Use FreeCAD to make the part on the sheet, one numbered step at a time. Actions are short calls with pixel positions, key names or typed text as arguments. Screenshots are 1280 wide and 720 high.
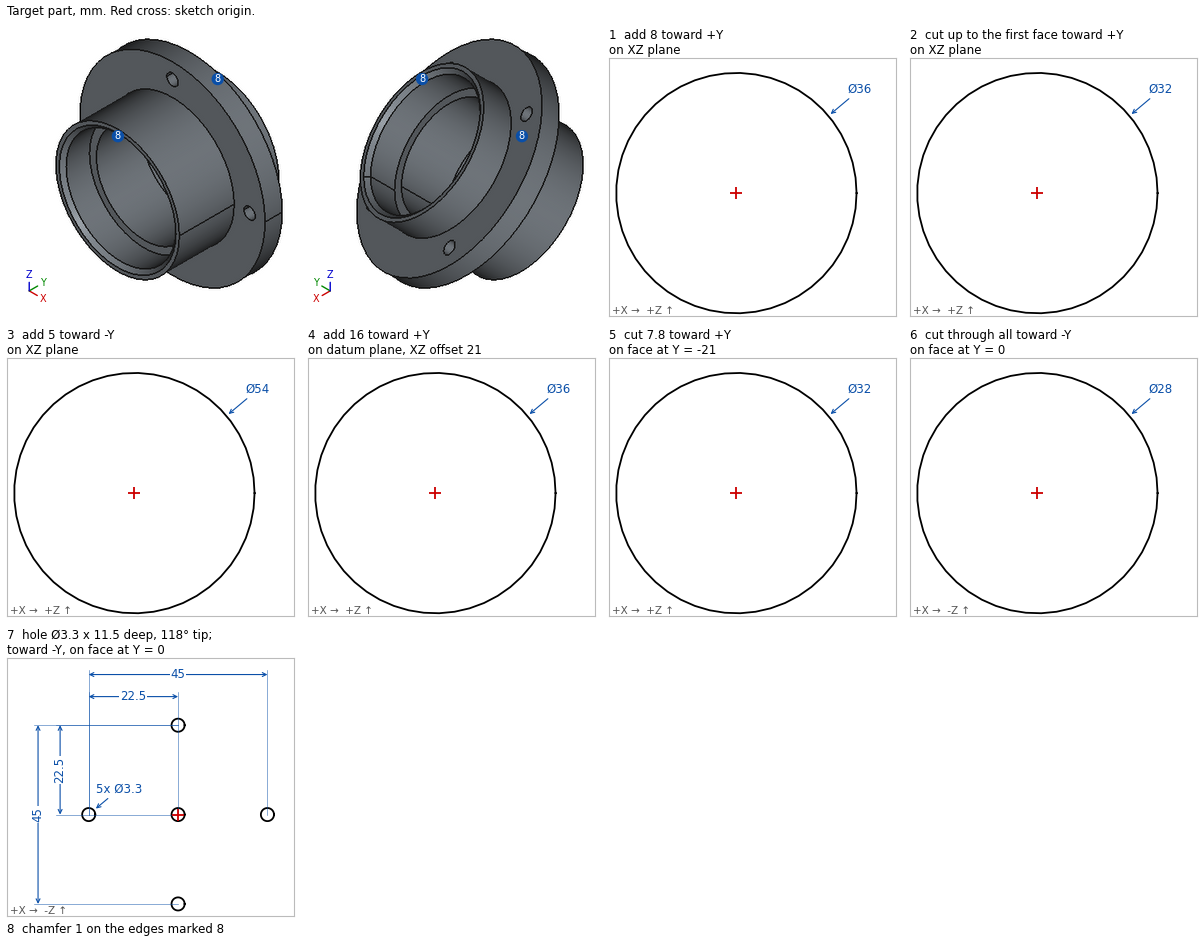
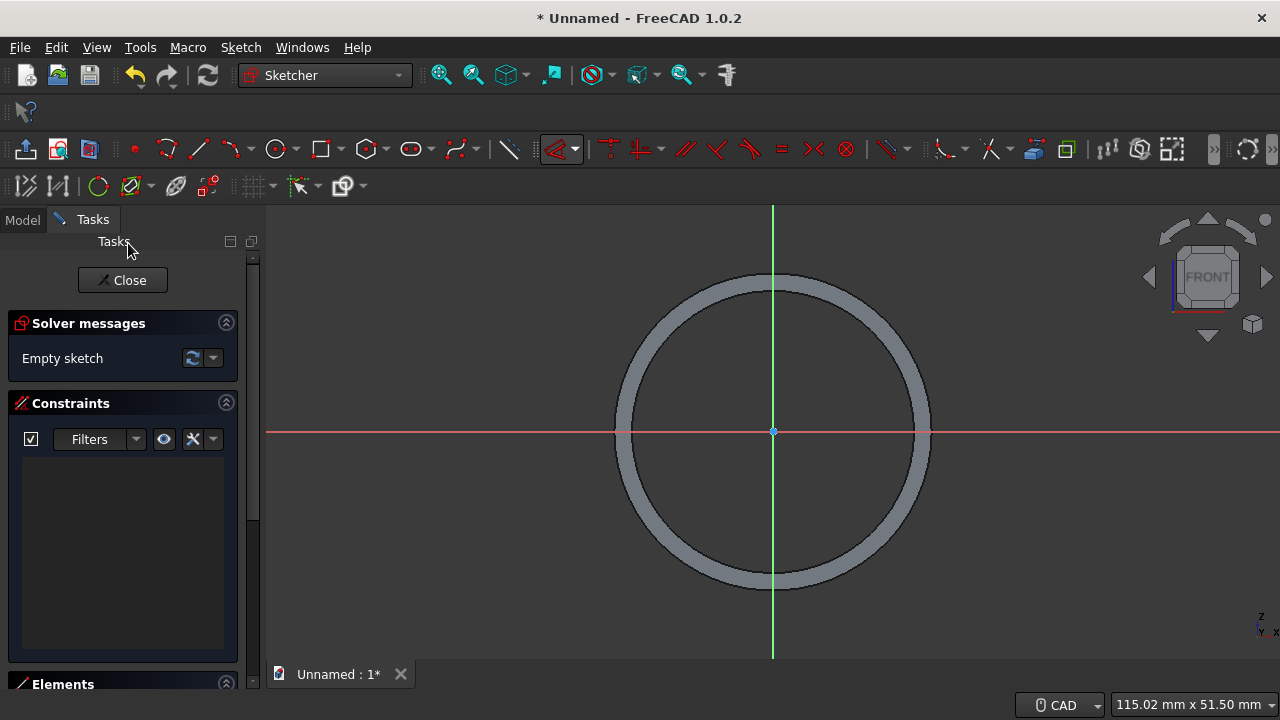
scroll(621, 432, down, 3)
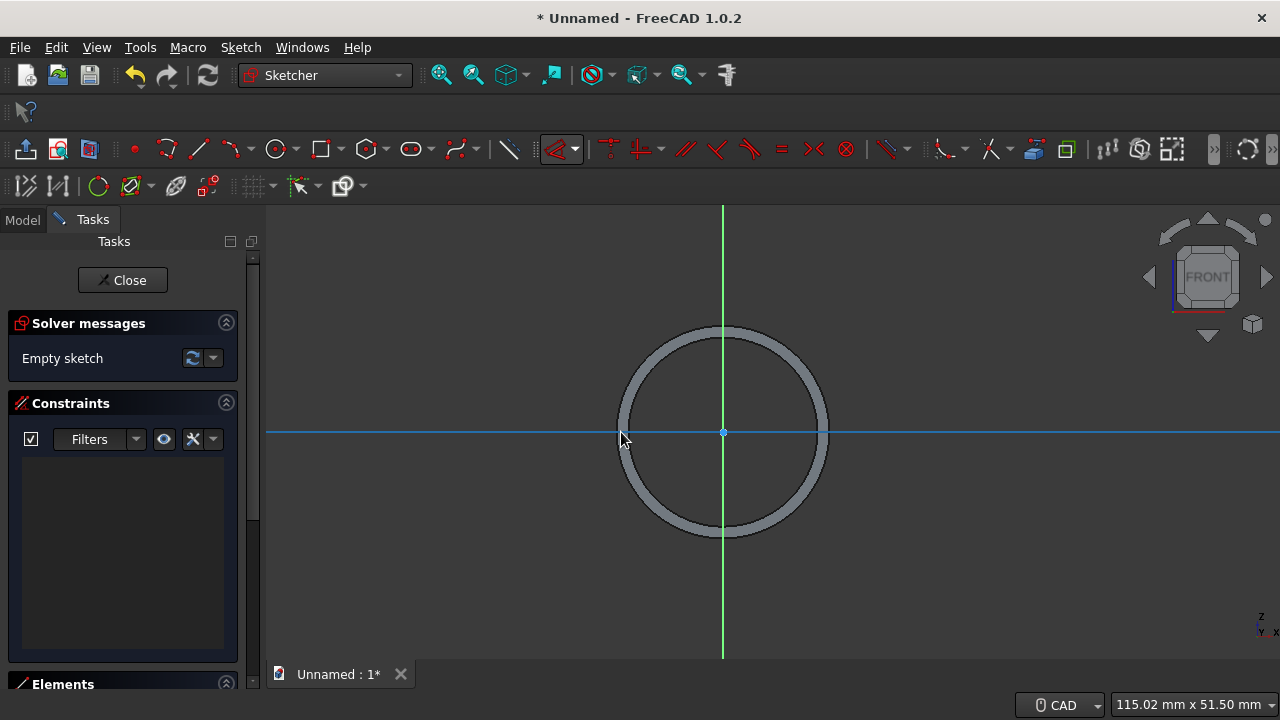
click(276, 150)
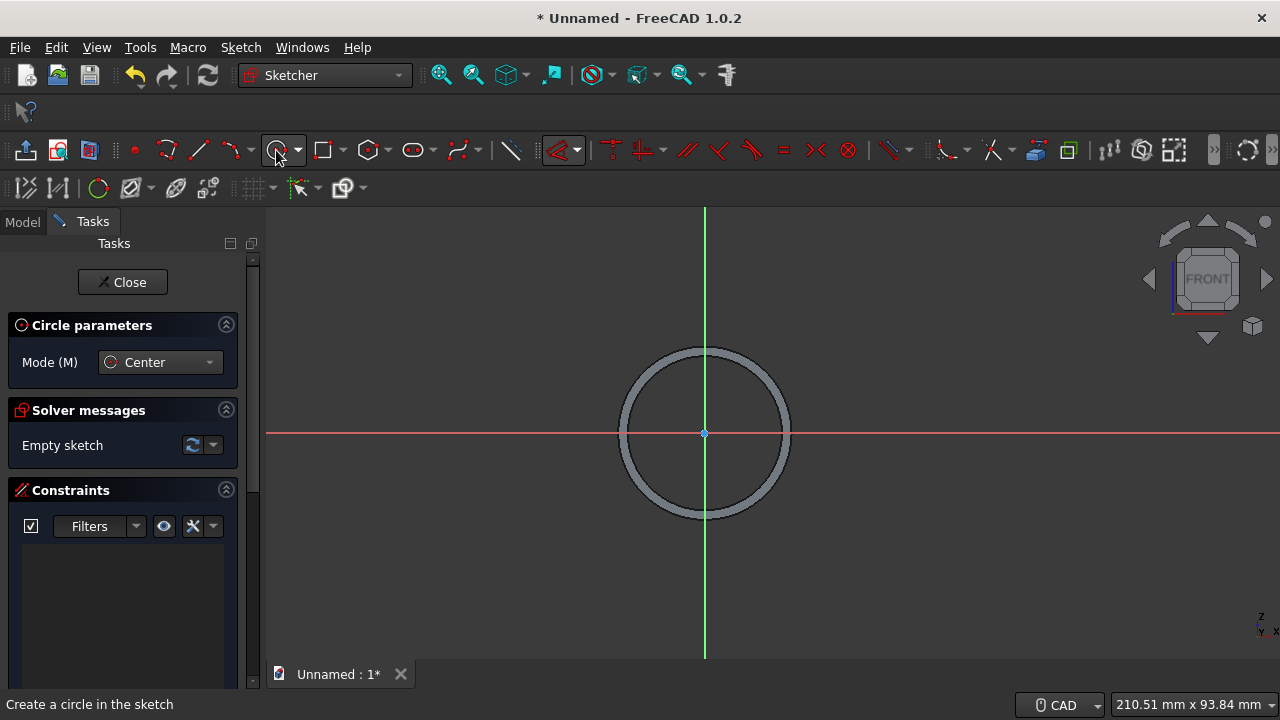
click(705, 433)
click(797, 341)
key(Escape)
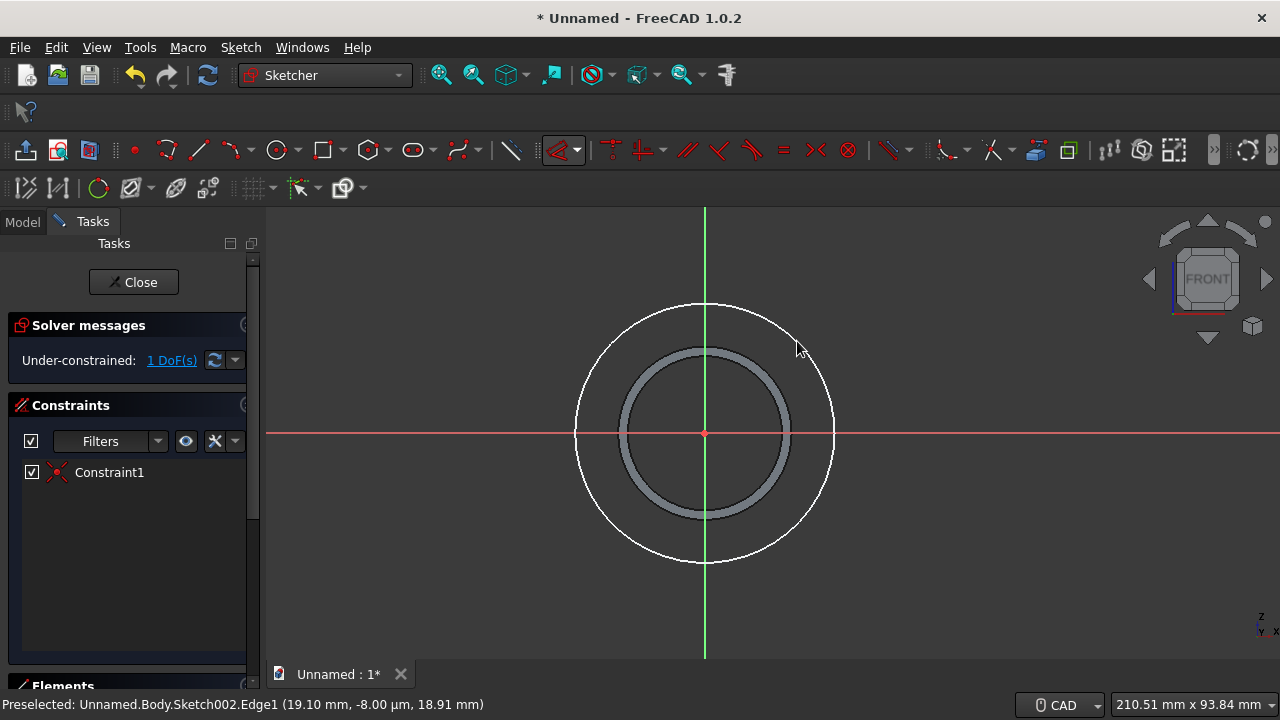
click(796, 341)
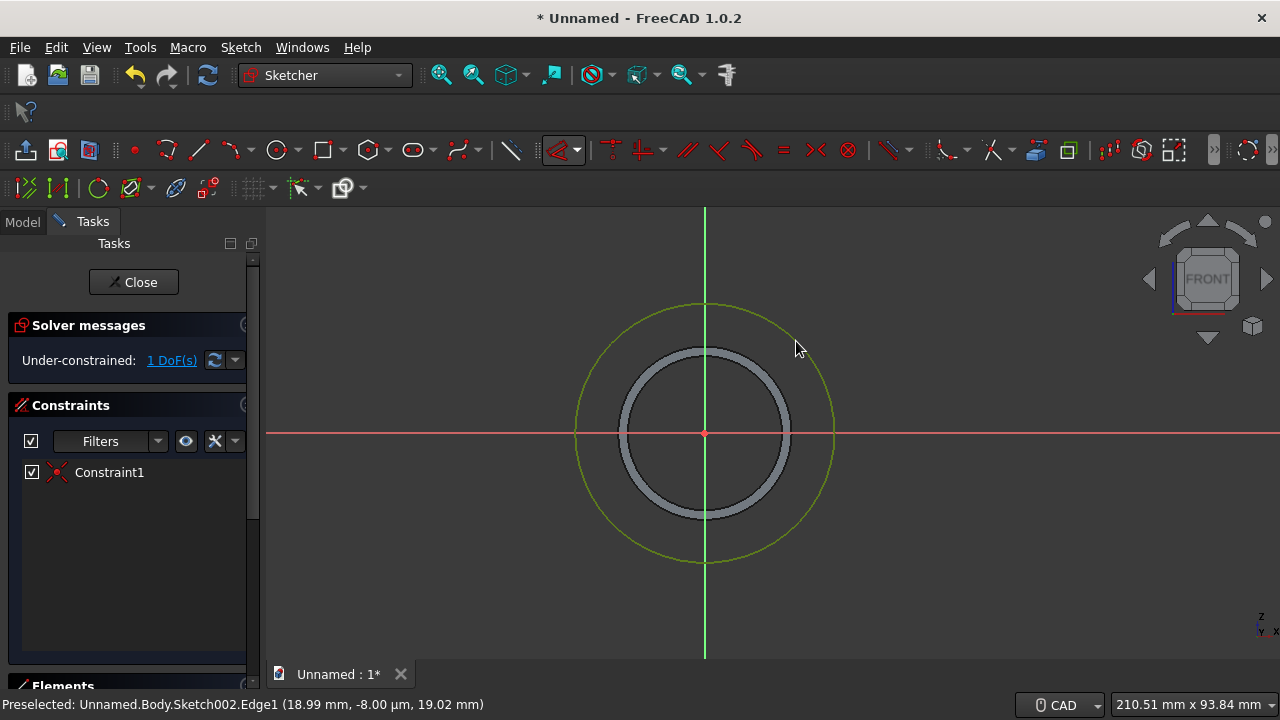
click(580, 150)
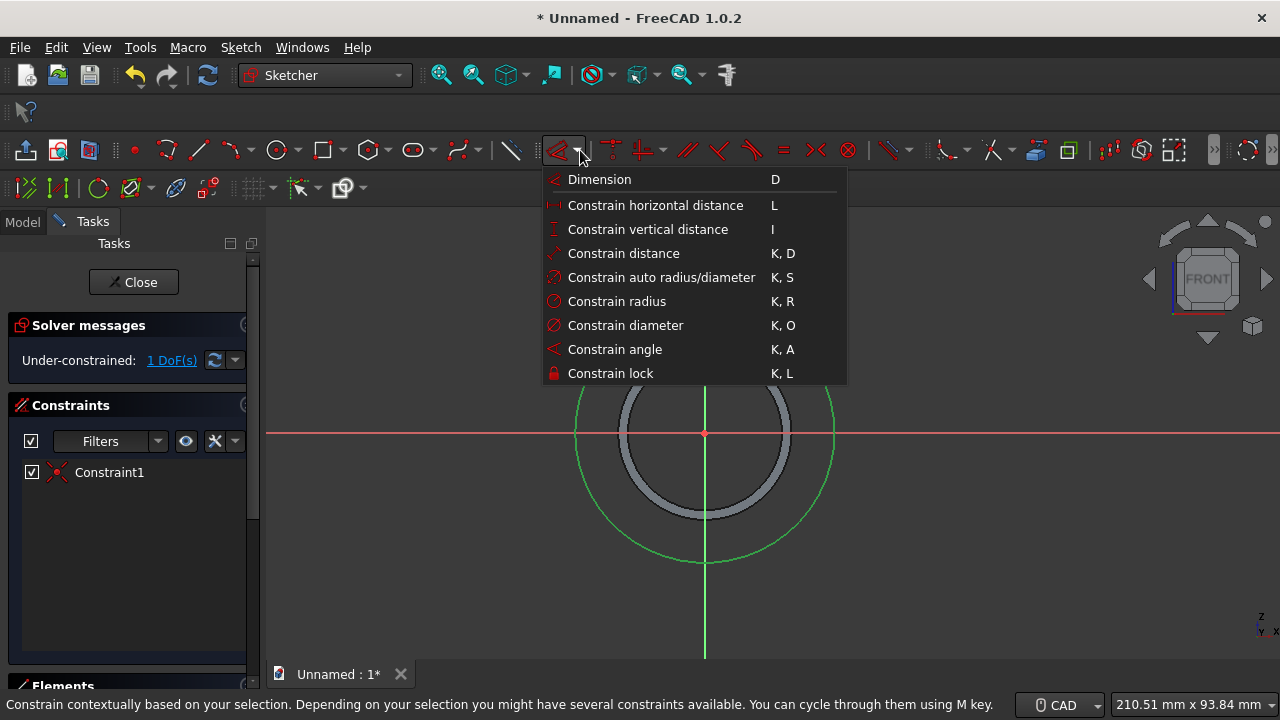
click(695, 325)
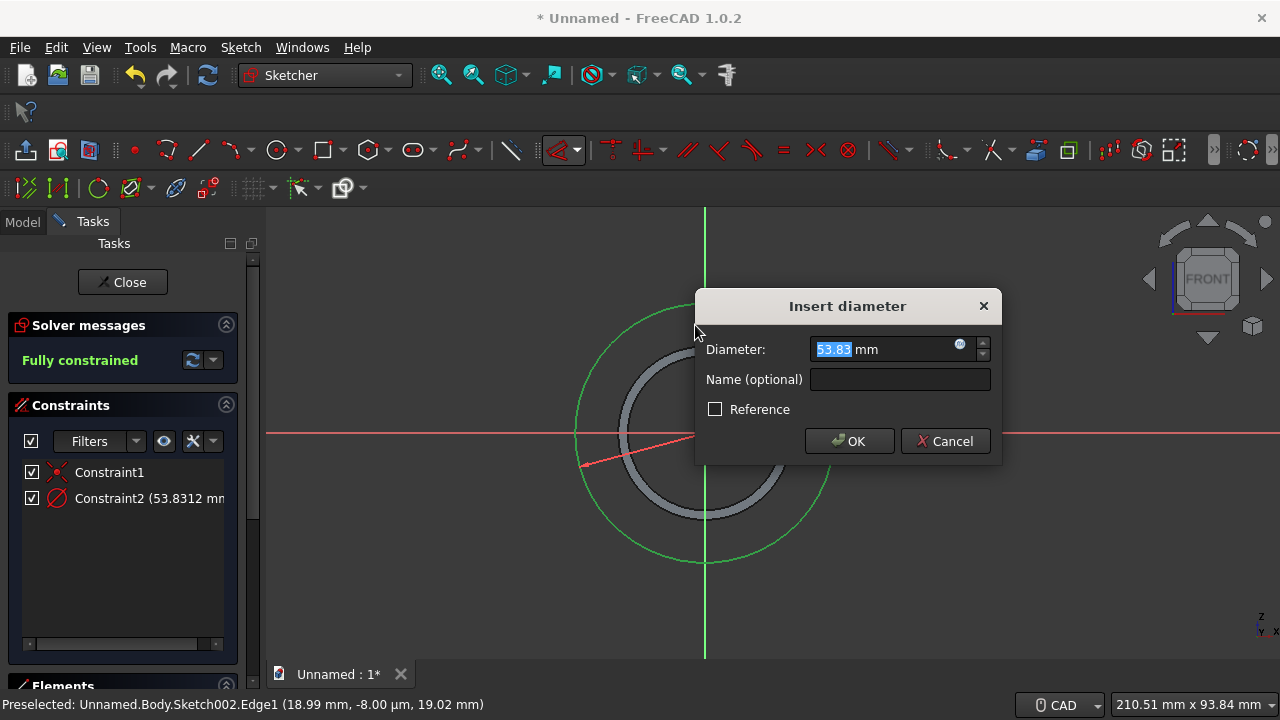
text(54)
key(Return)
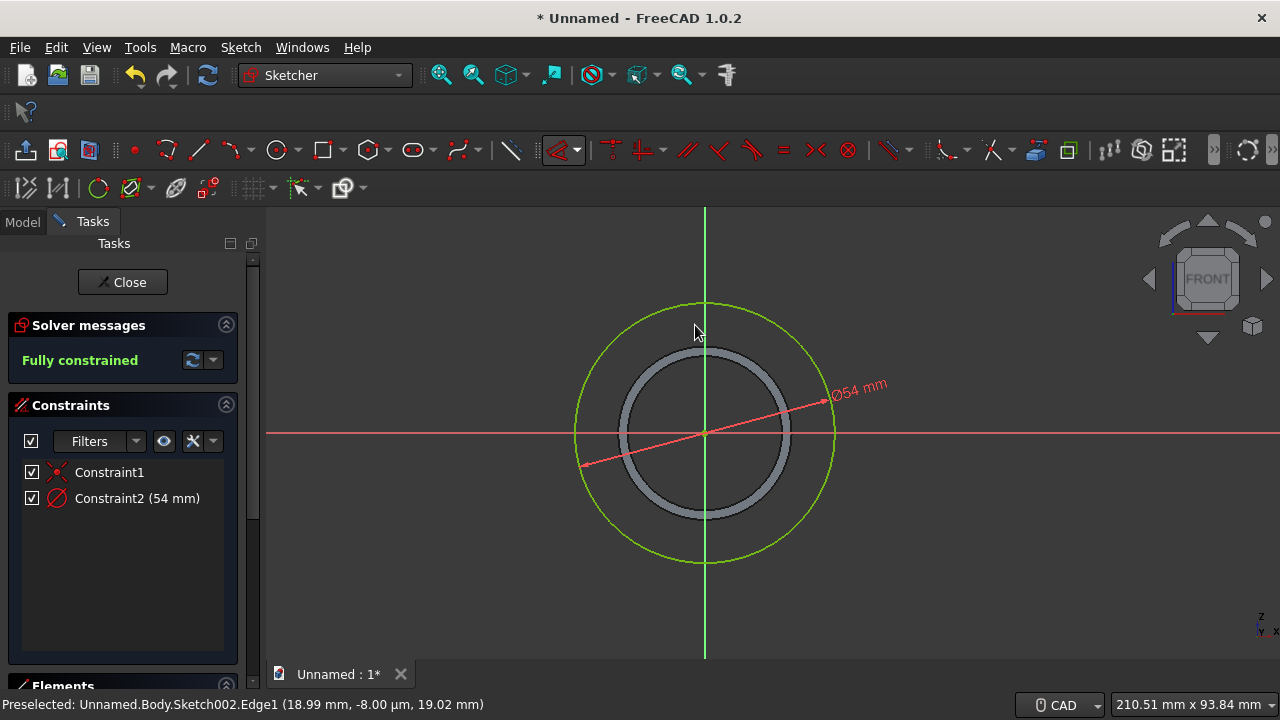
click(123, 282)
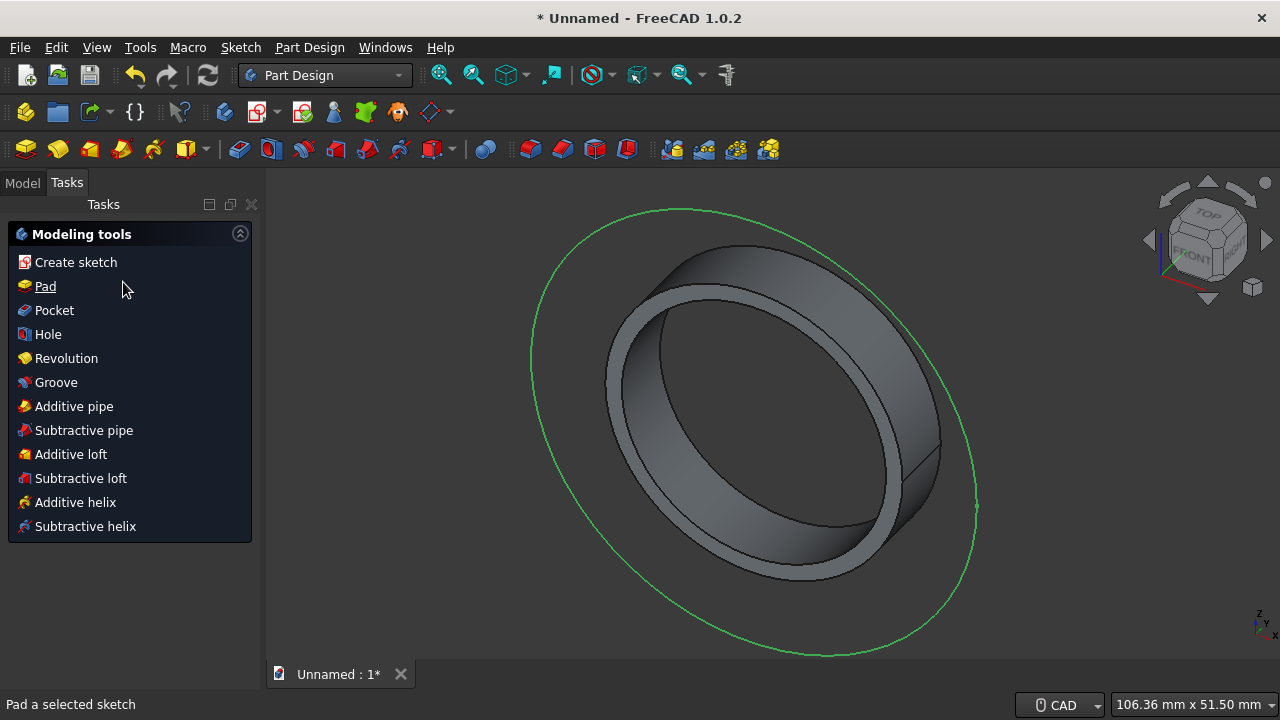
click(26, 150)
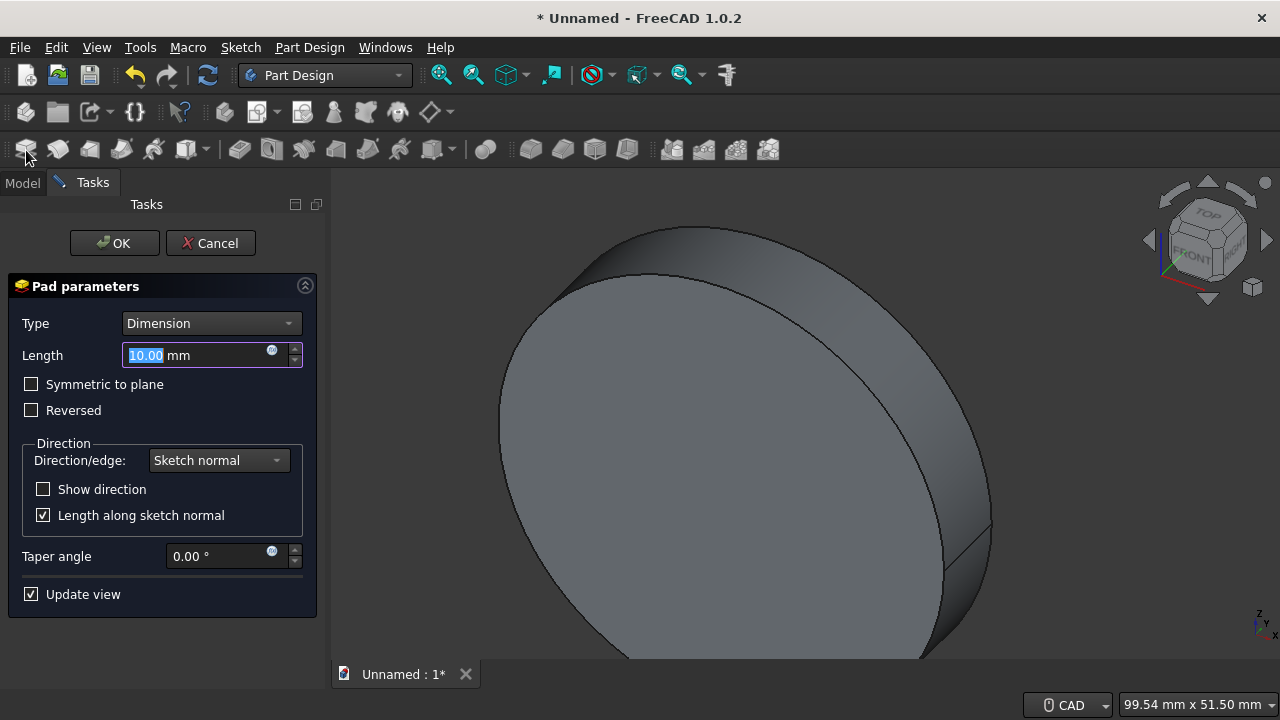
text(5)
key(Tab)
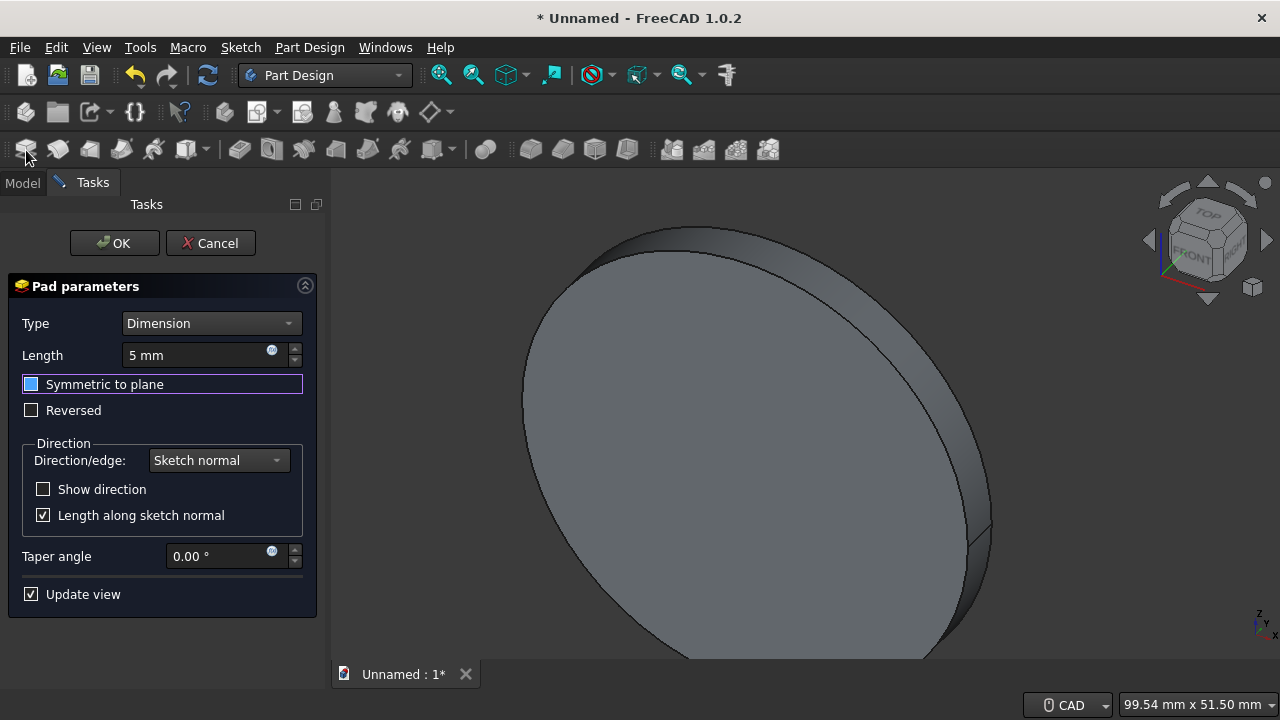
click(115, 243)